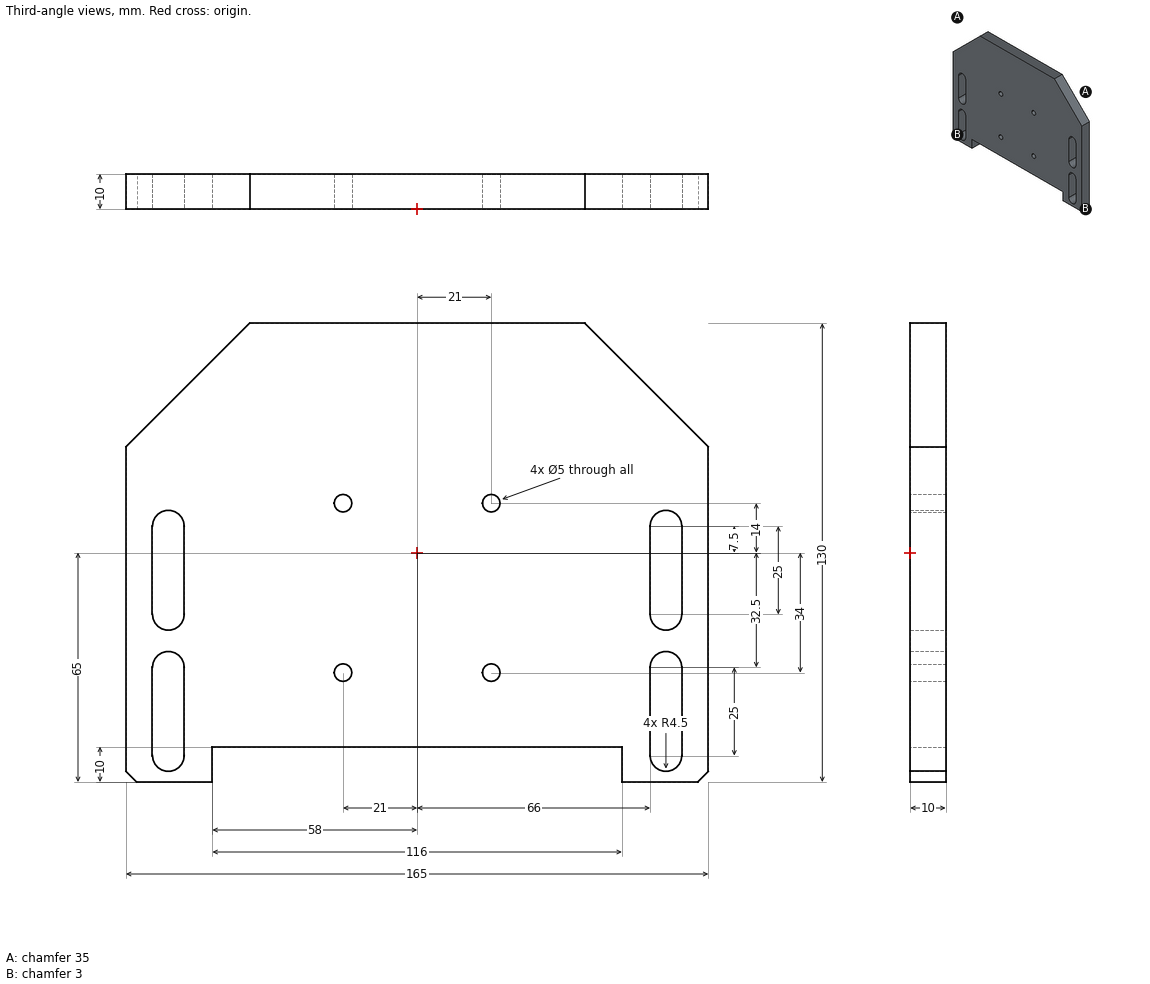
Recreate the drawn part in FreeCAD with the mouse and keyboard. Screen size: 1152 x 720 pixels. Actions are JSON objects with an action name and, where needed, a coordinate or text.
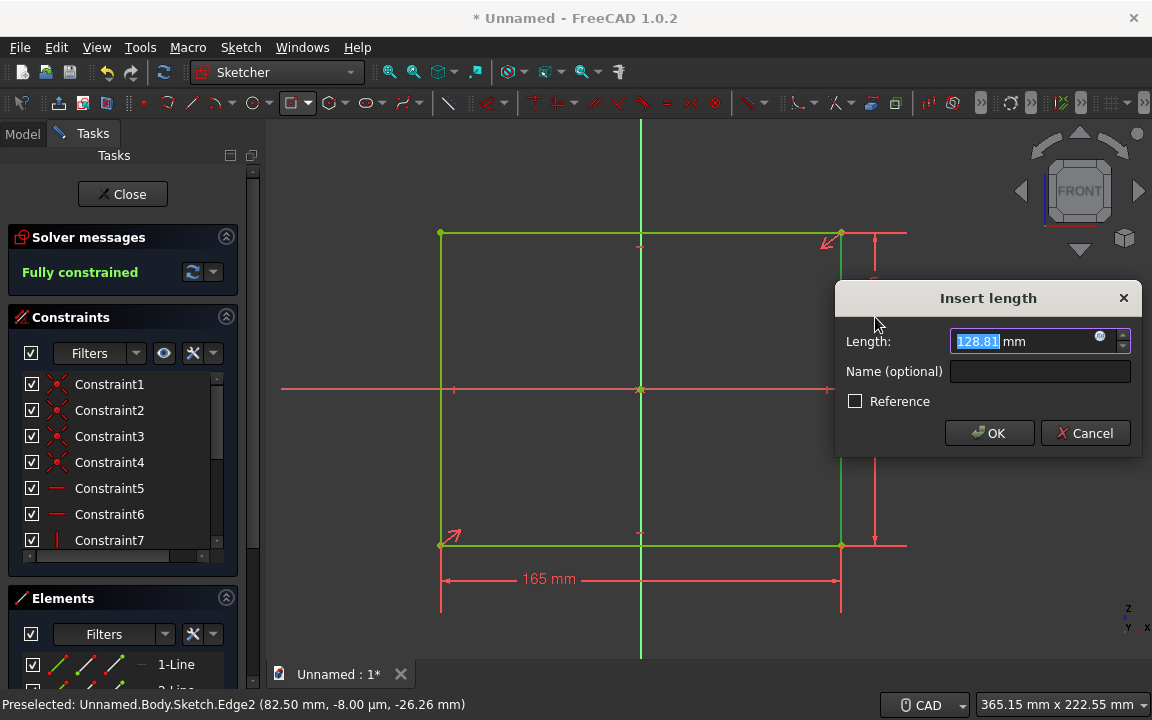
{"action": "type", "text": "130"}
{"action": "key", "text": "Return"}
{"action": "key", "text": "Escape"}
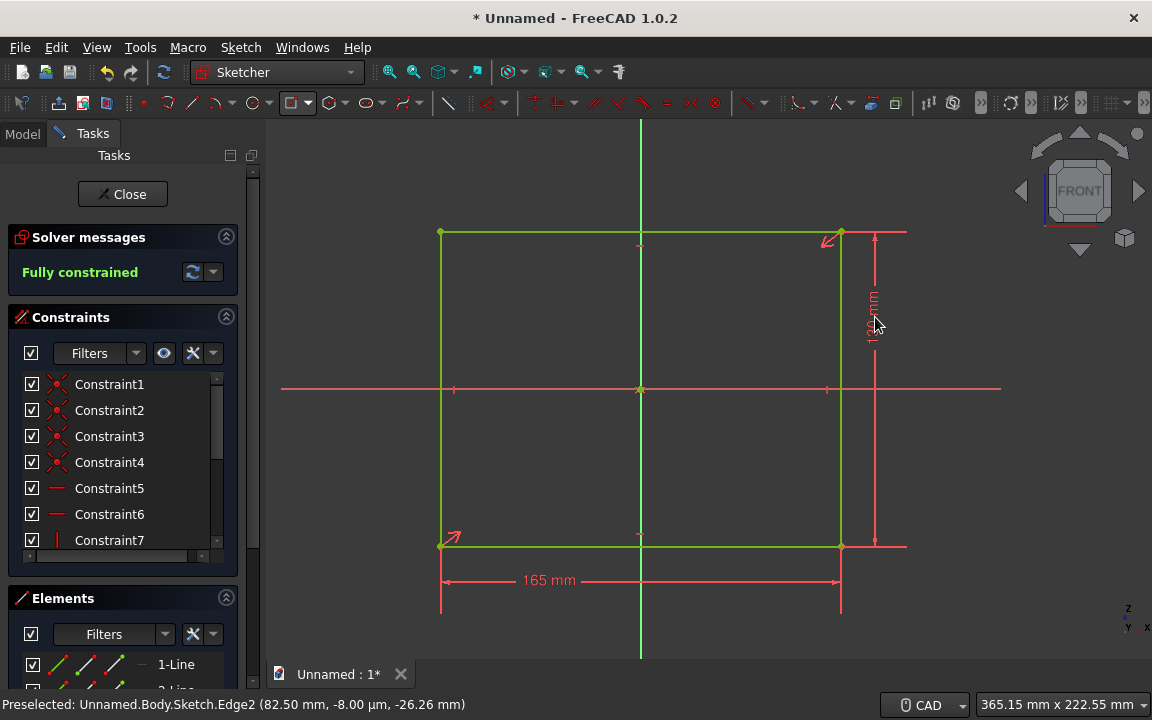
{"action": "left_click", "coordinate": [123, 194]}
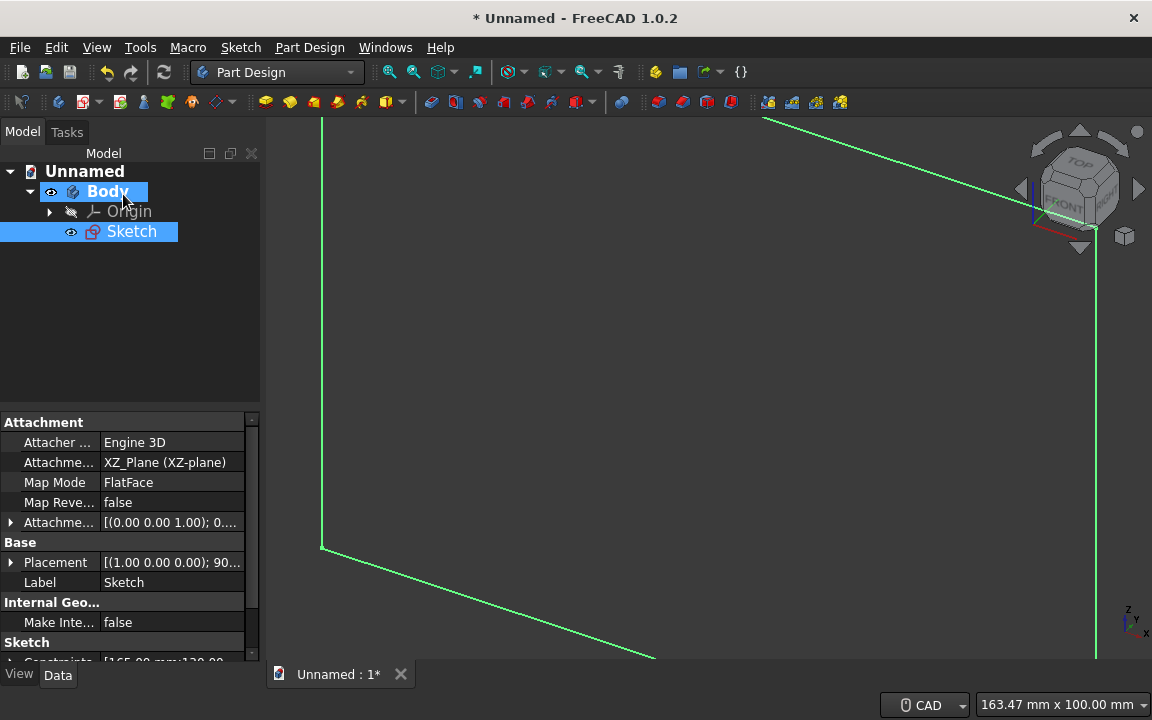
{"action": "left_click", "coordinate": [266, 102]}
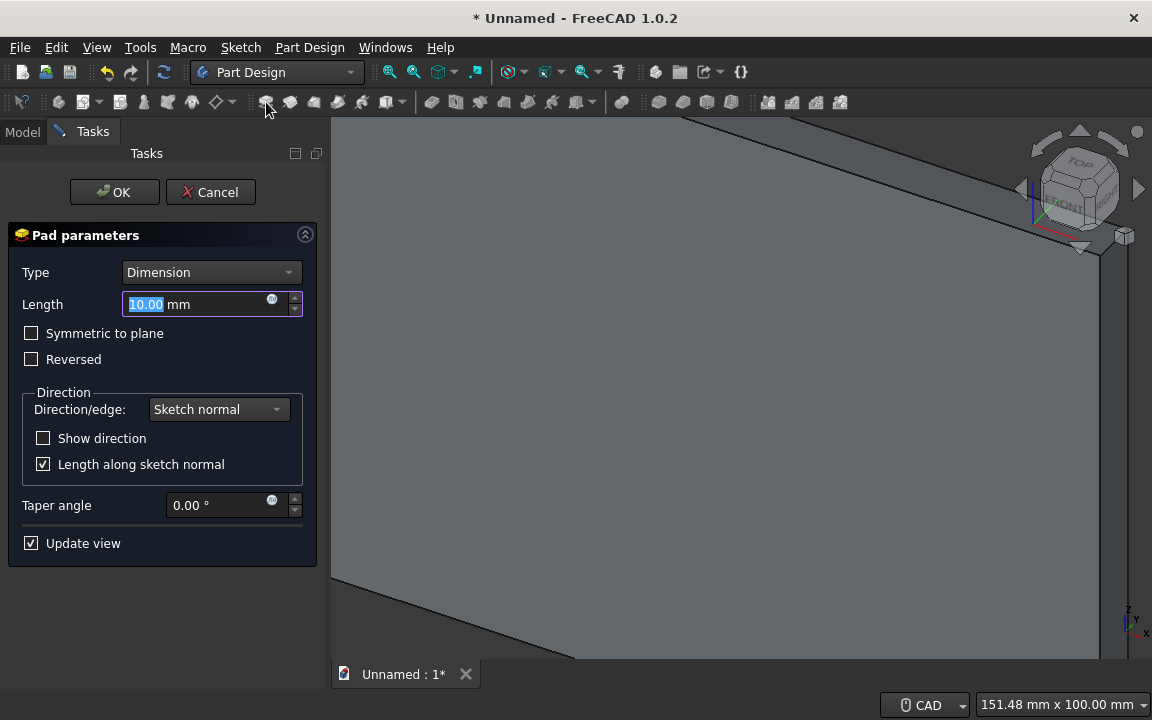
{"action": "type", "text": "10"}
{"action": "key", "text": "Tab"}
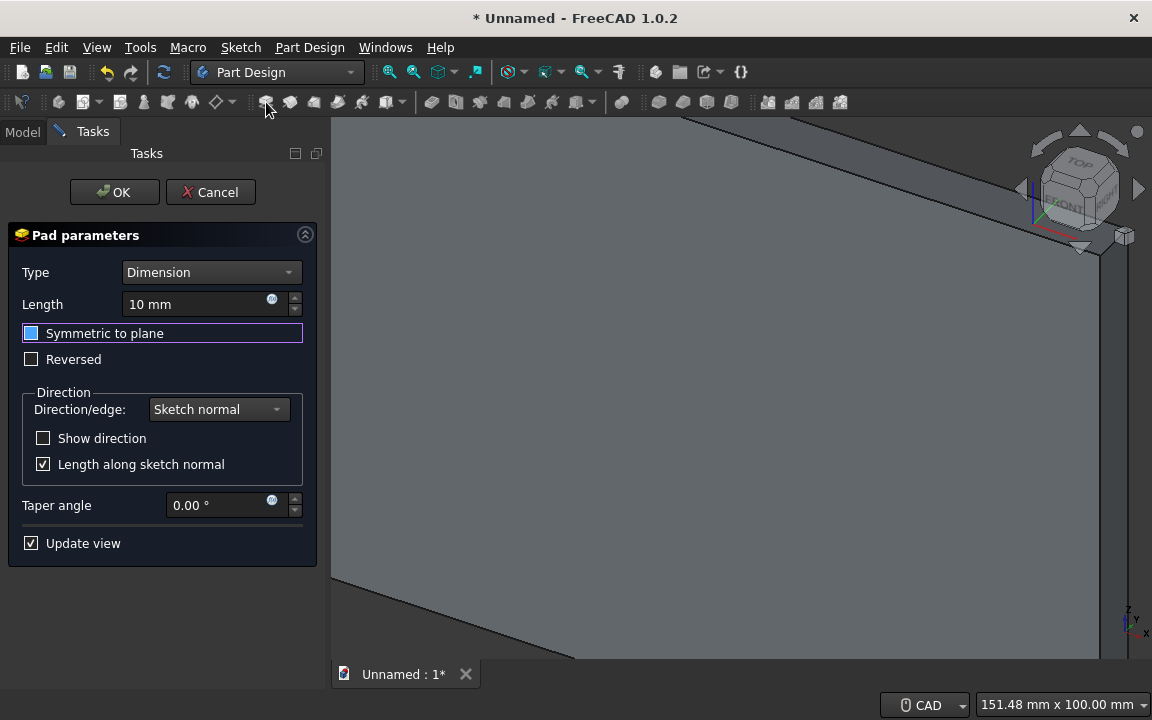
{"action": "left_click", "coordinate": [30, 359]}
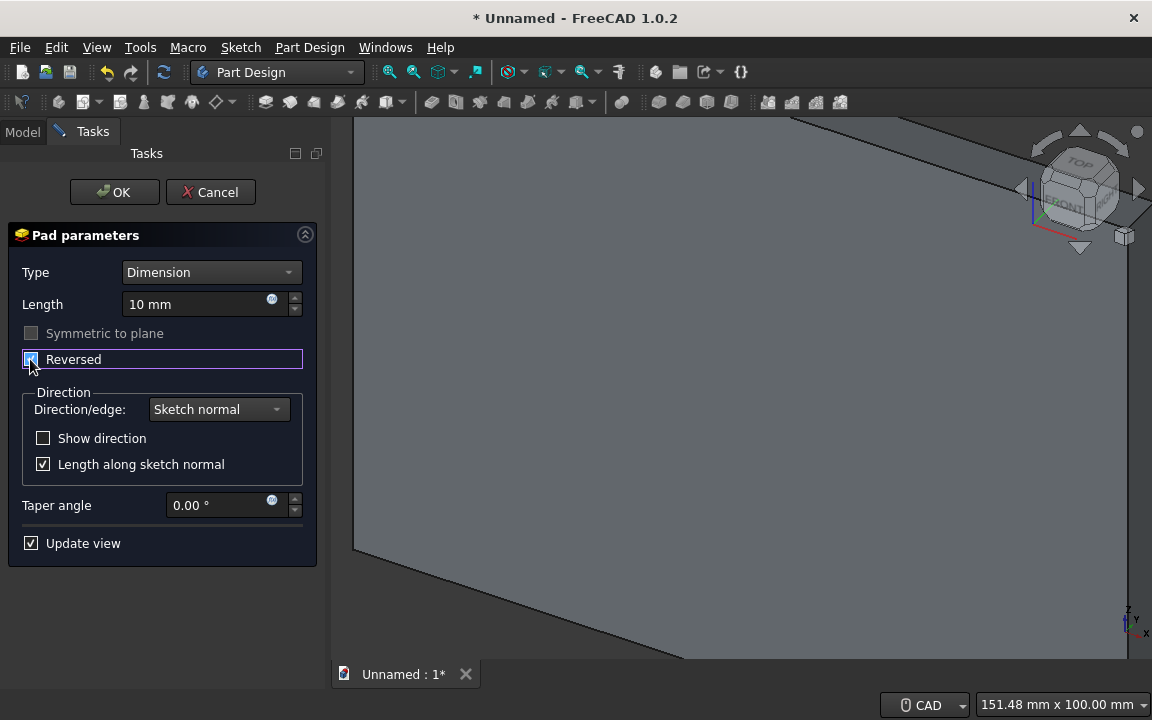
{"action": "left_click", "coordinate": [115, 192]}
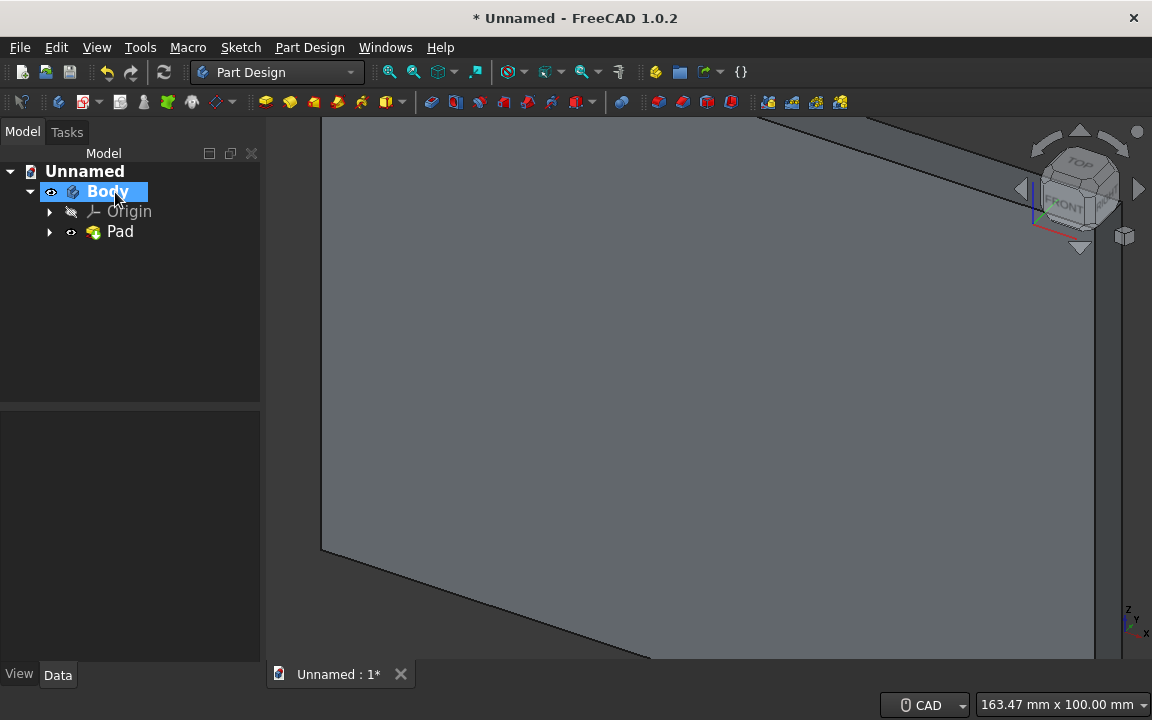
{"action": "left_click", "coordinate": [390, 72]}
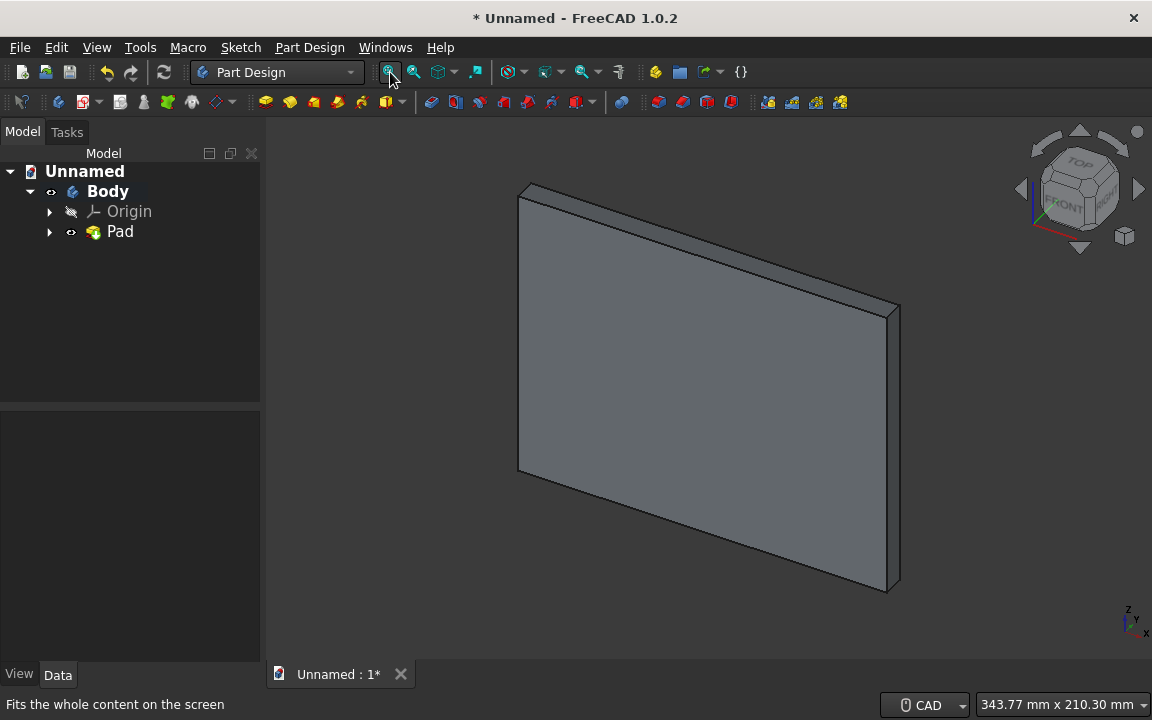
{"action": "key", "text": "4"}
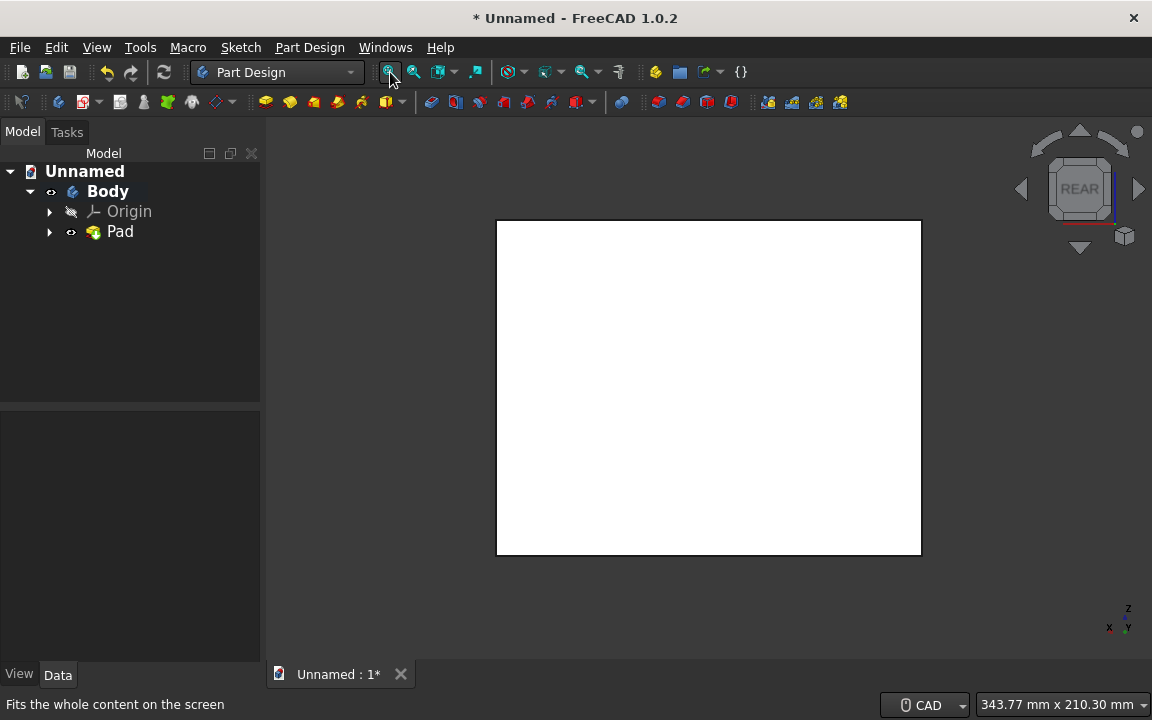
{"action": "left_click", "coordinate": [709, 387]}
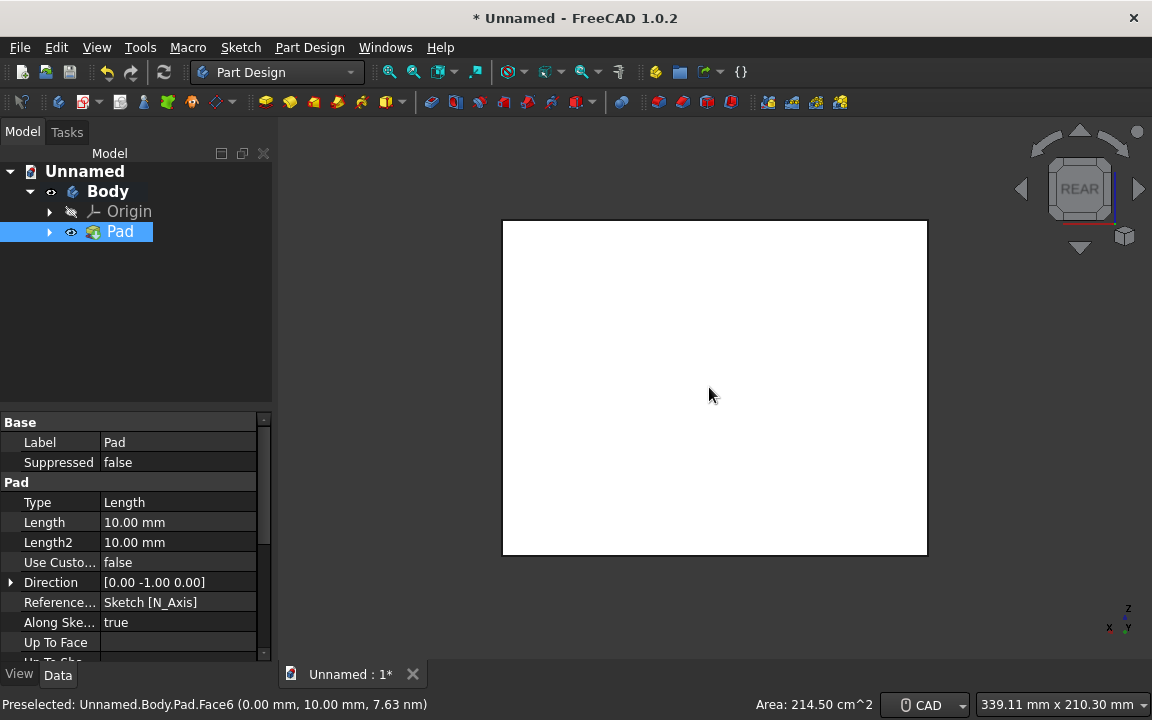
{"action": "left_click", "coordinate": [84, 102]}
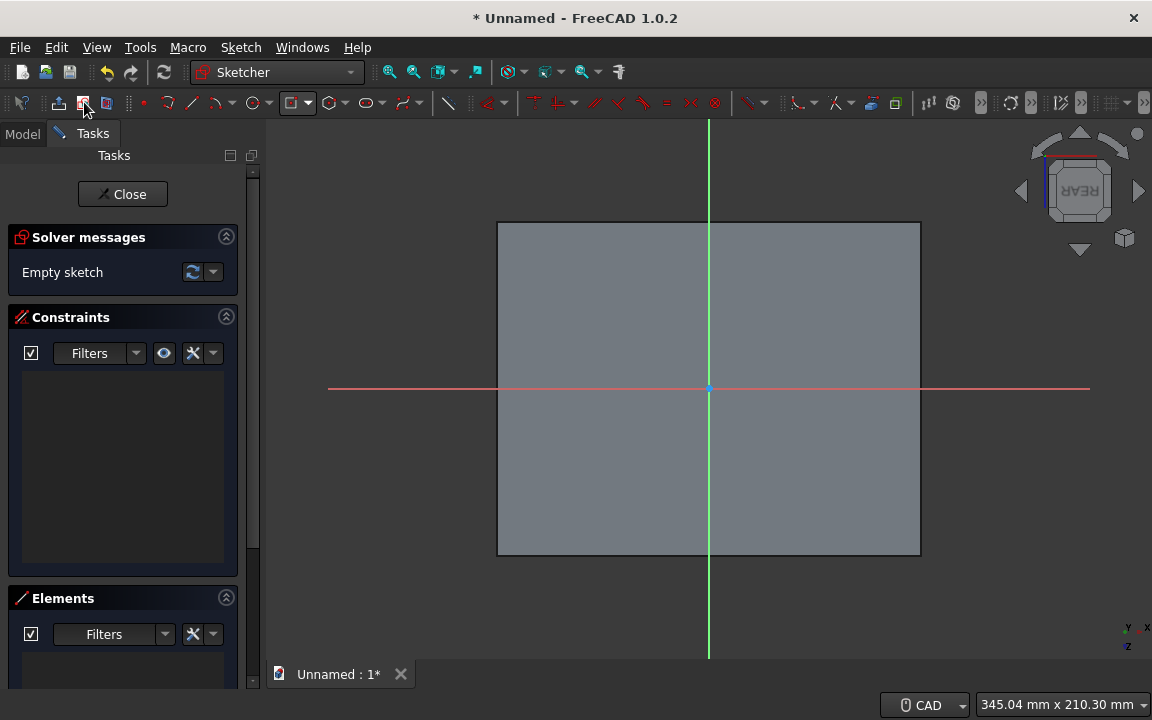
{"action": "scroll", "coordinate": [848, 147], "scroll_direction": "up", "scroll_amount": 2}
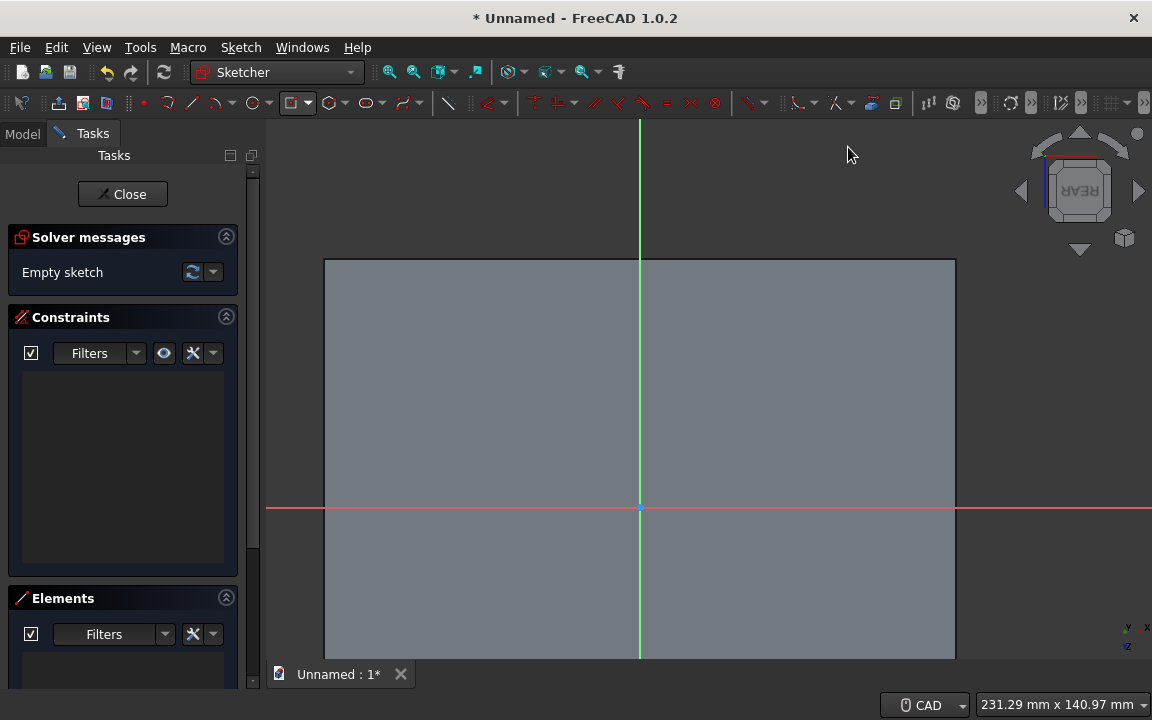
{"action": "key", "text": "g r"}